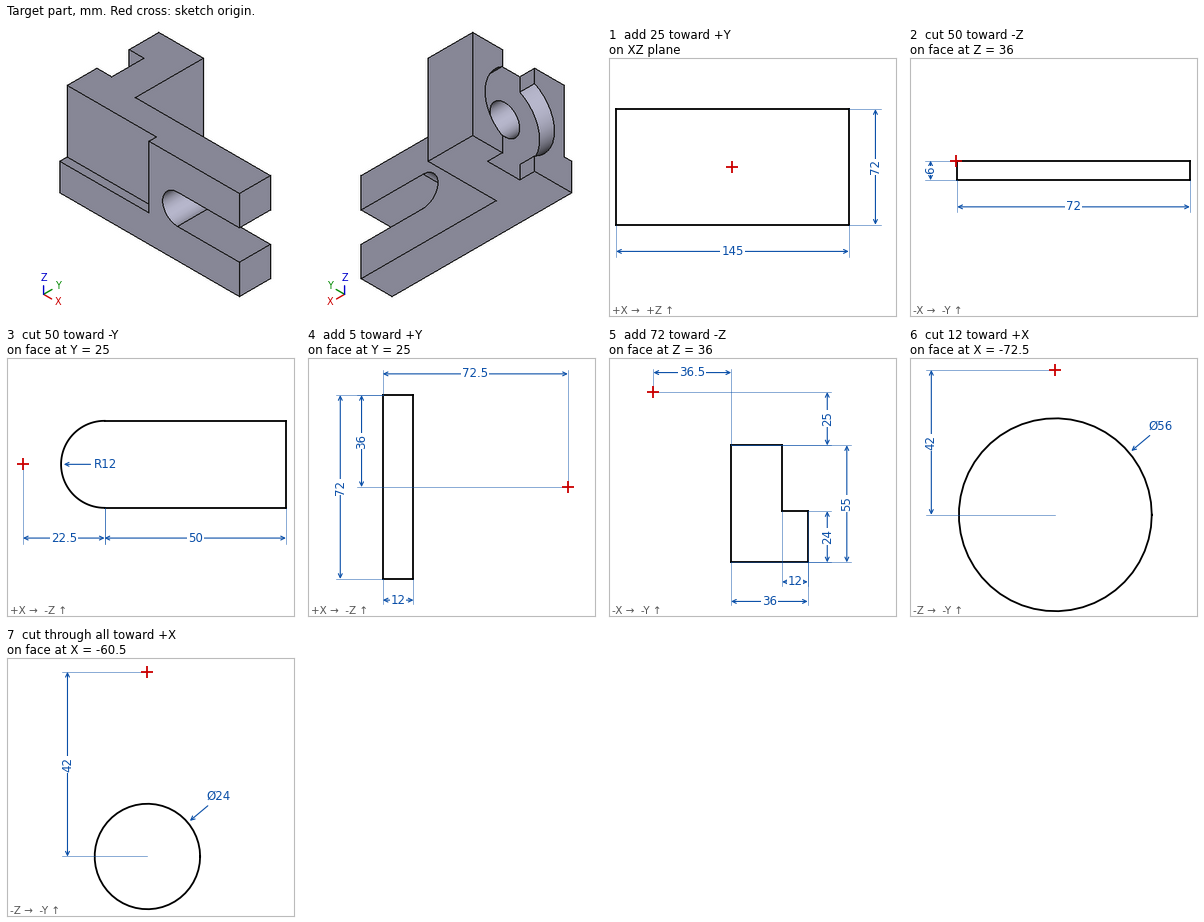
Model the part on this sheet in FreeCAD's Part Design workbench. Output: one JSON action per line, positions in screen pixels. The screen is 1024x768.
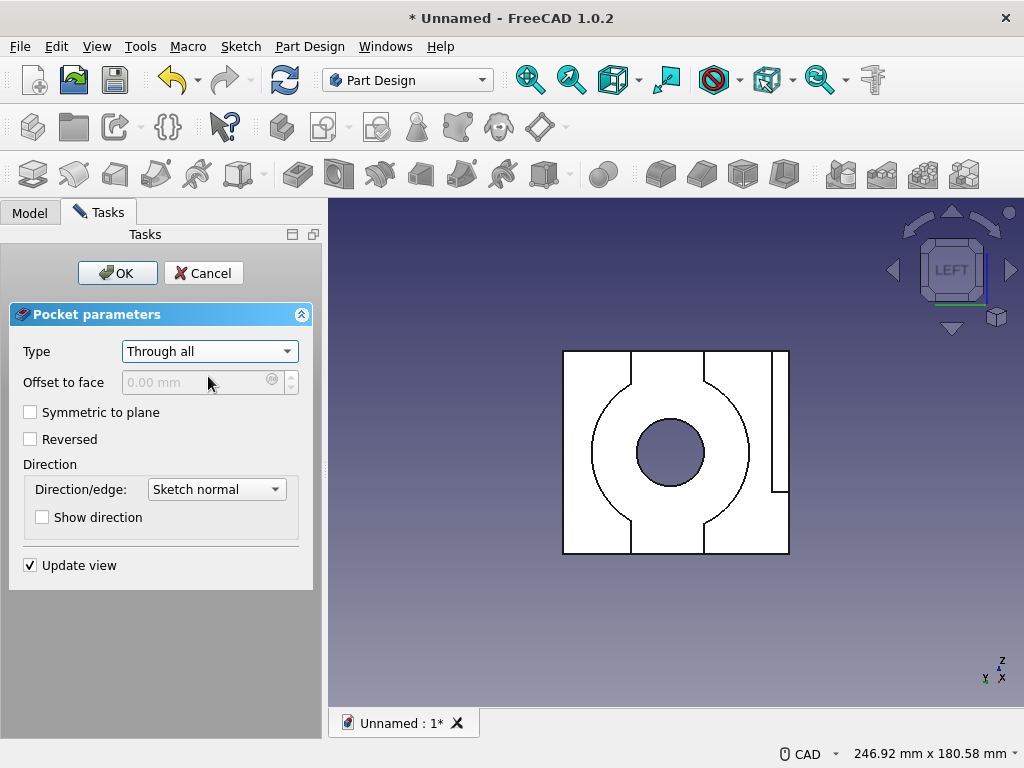
{"action": "left_click", "coordinate": [118, 273]}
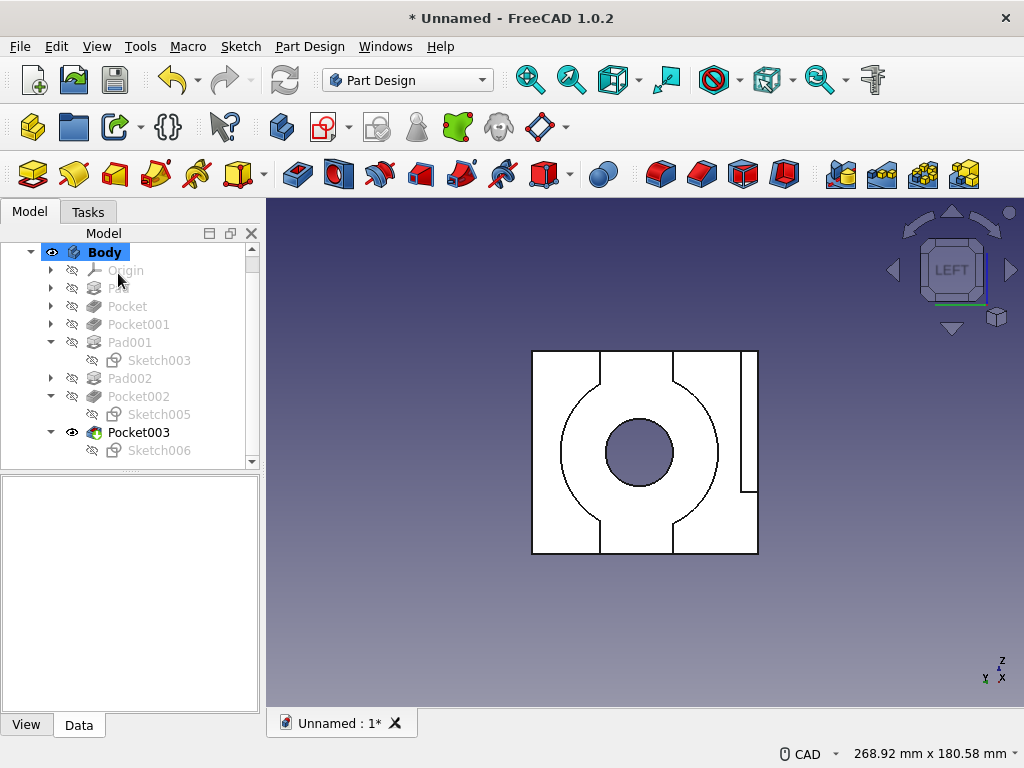
{"action": "key", "text": "0"}